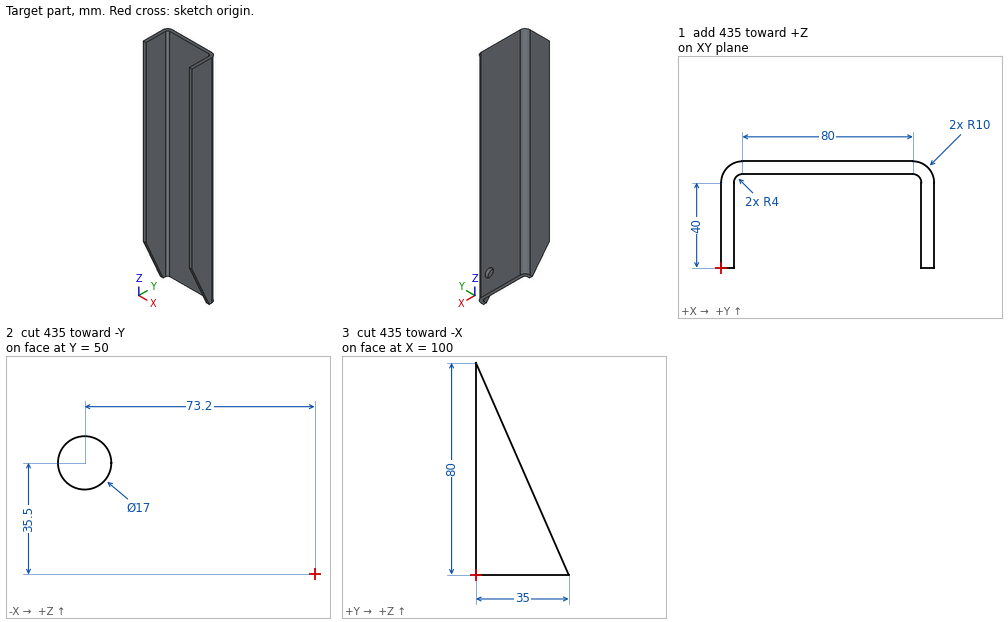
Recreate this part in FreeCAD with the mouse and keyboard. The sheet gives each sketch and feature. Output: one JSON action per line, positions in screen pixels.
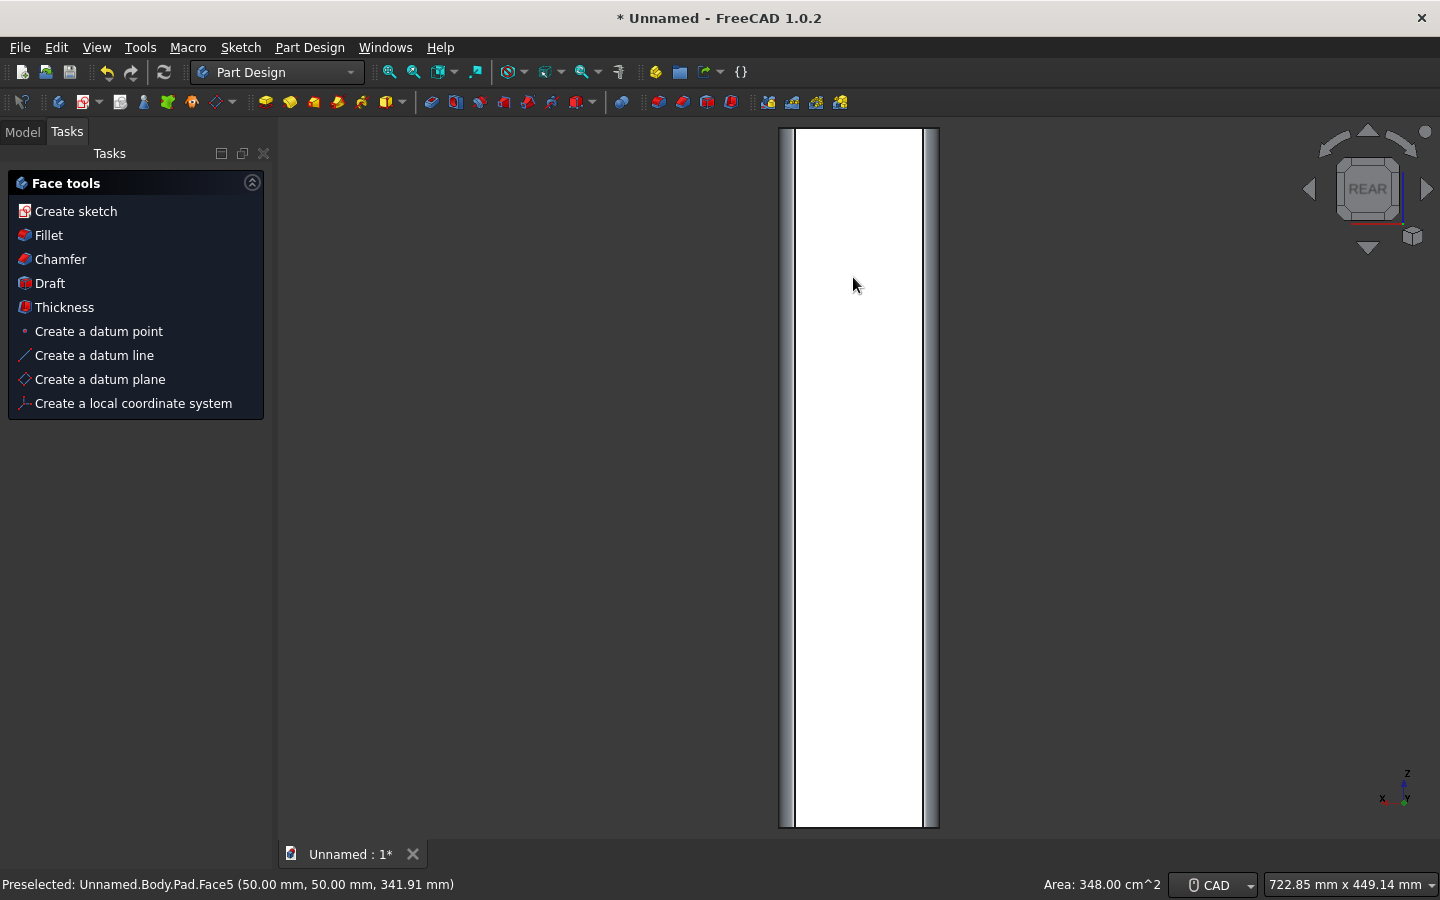
{"action": "left_click", "coordinate": [84, 102]}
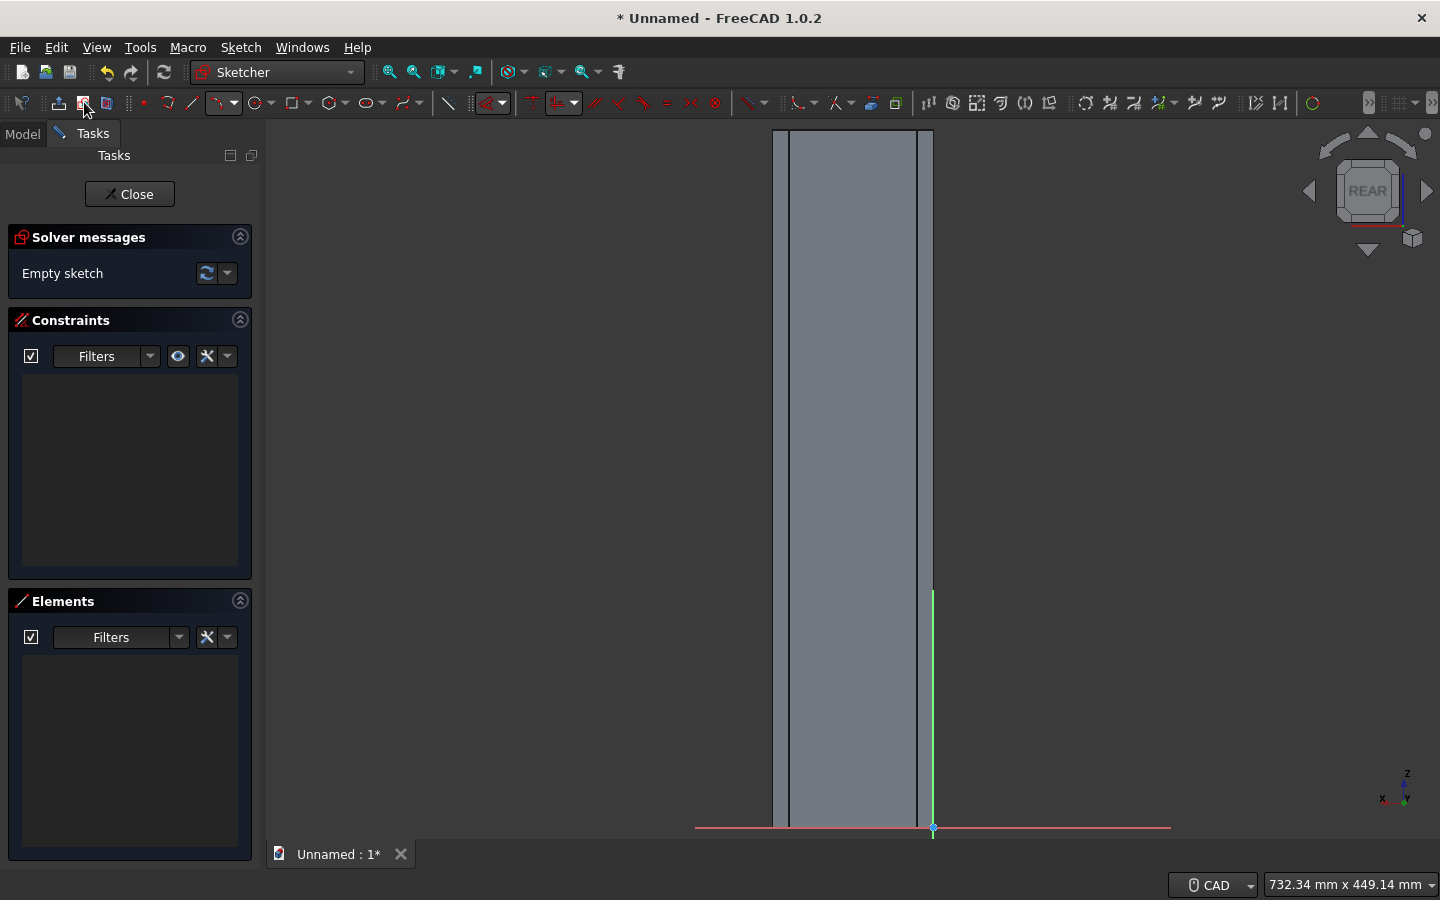
{"action": "scroll", "coordinate": [818, 790], "scroll_direction": "up", "scroll_amount": 14}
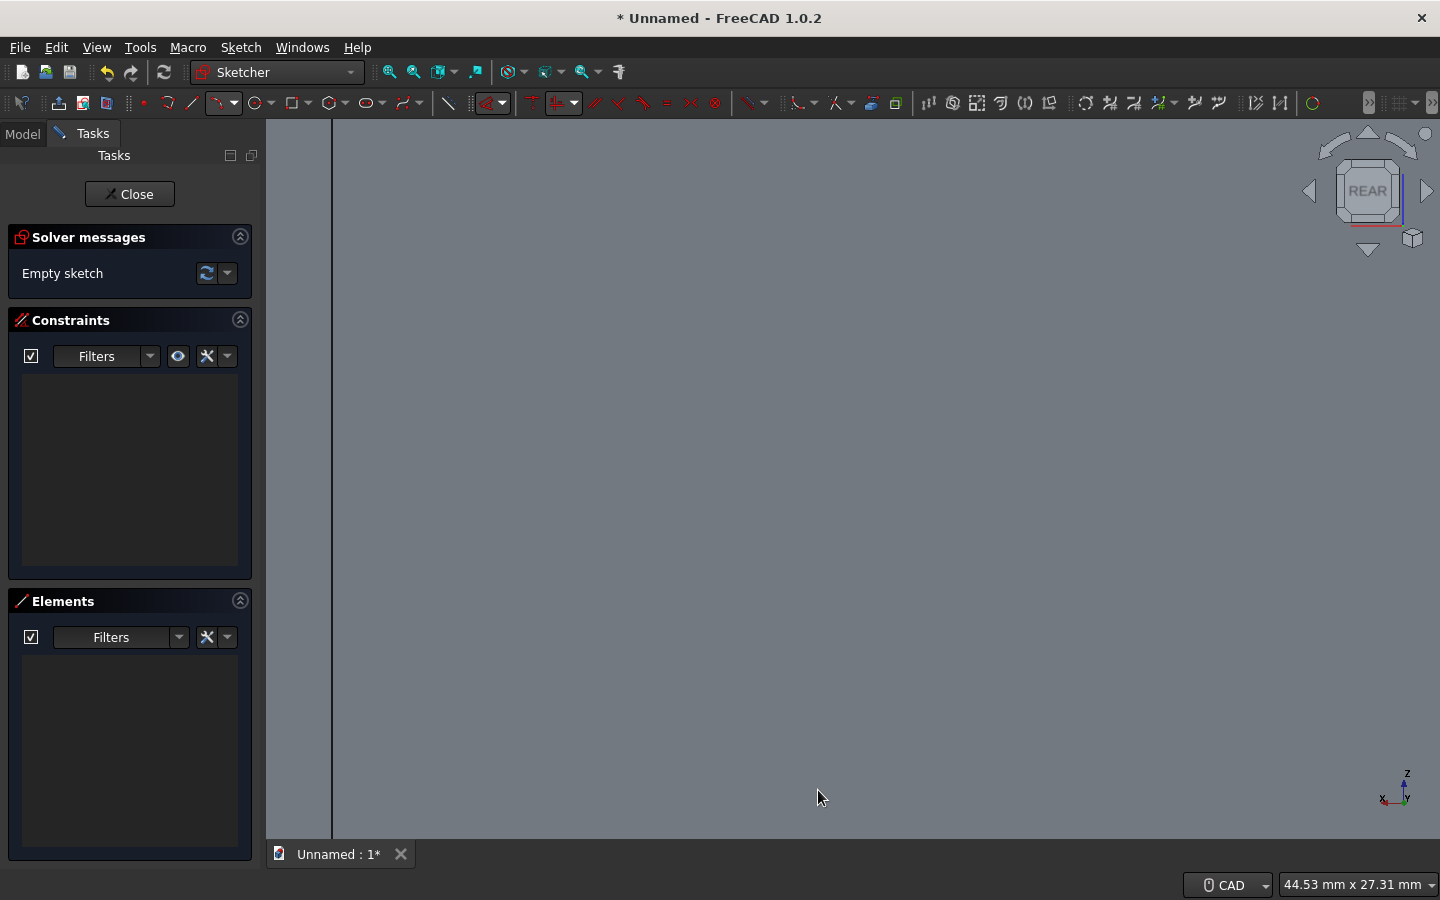
{"action": "left_click", "coordinate": [256, 104]}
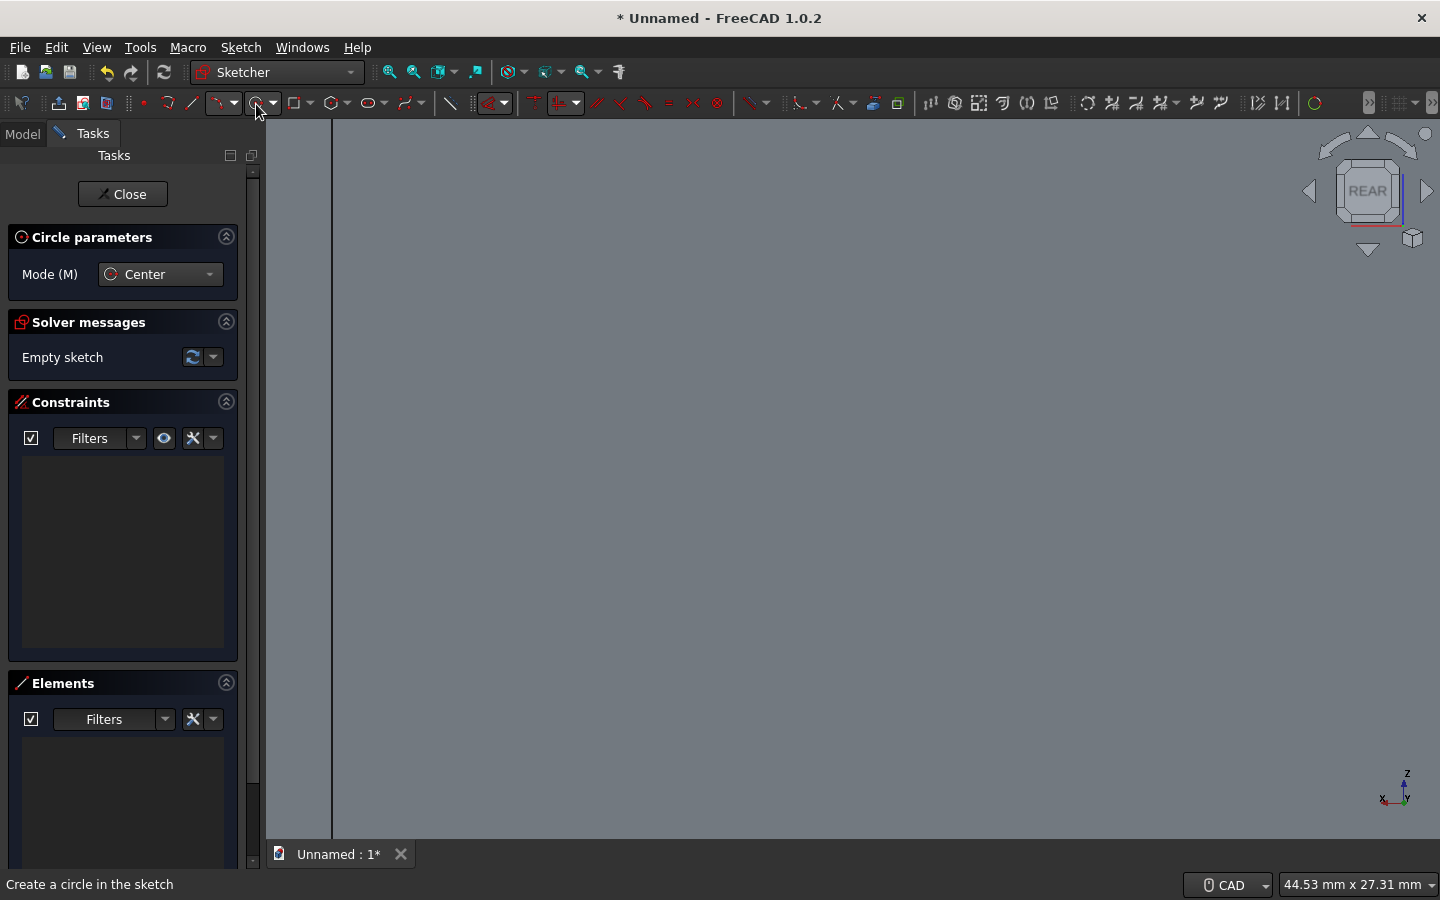
{"action": "left_click", "coordinate": [775, 459]}
{"action": "mouse_move", "coordinate": [933, 301]}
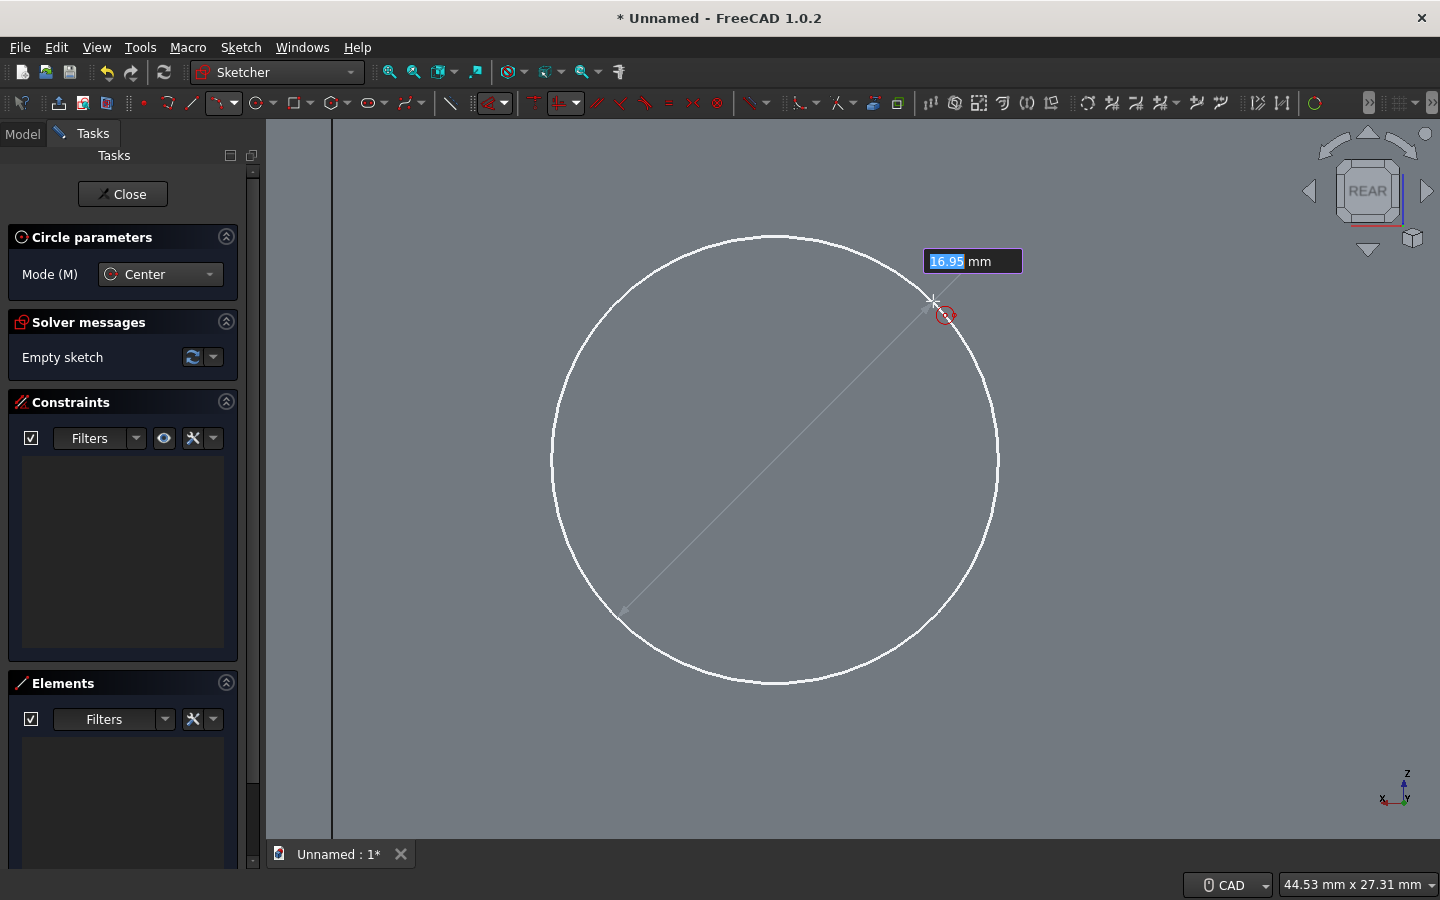
{"action": "type", "text": "17"}
{"action": "key", "text": "Return"}
{"action": "key", "text": "Escape"}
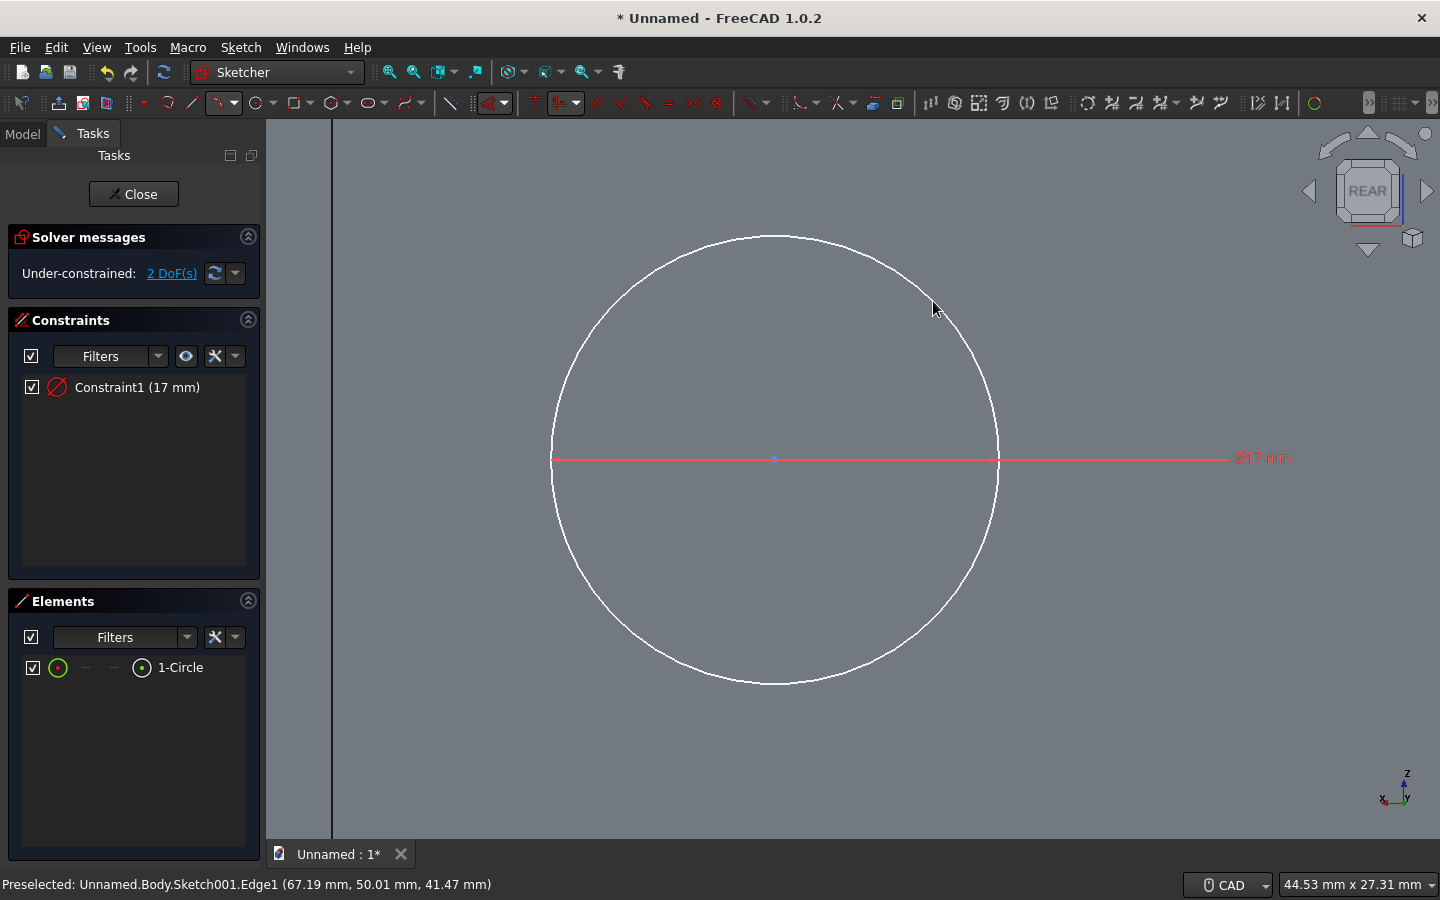
{"action": "left_click", "coordinate": [775, 460]}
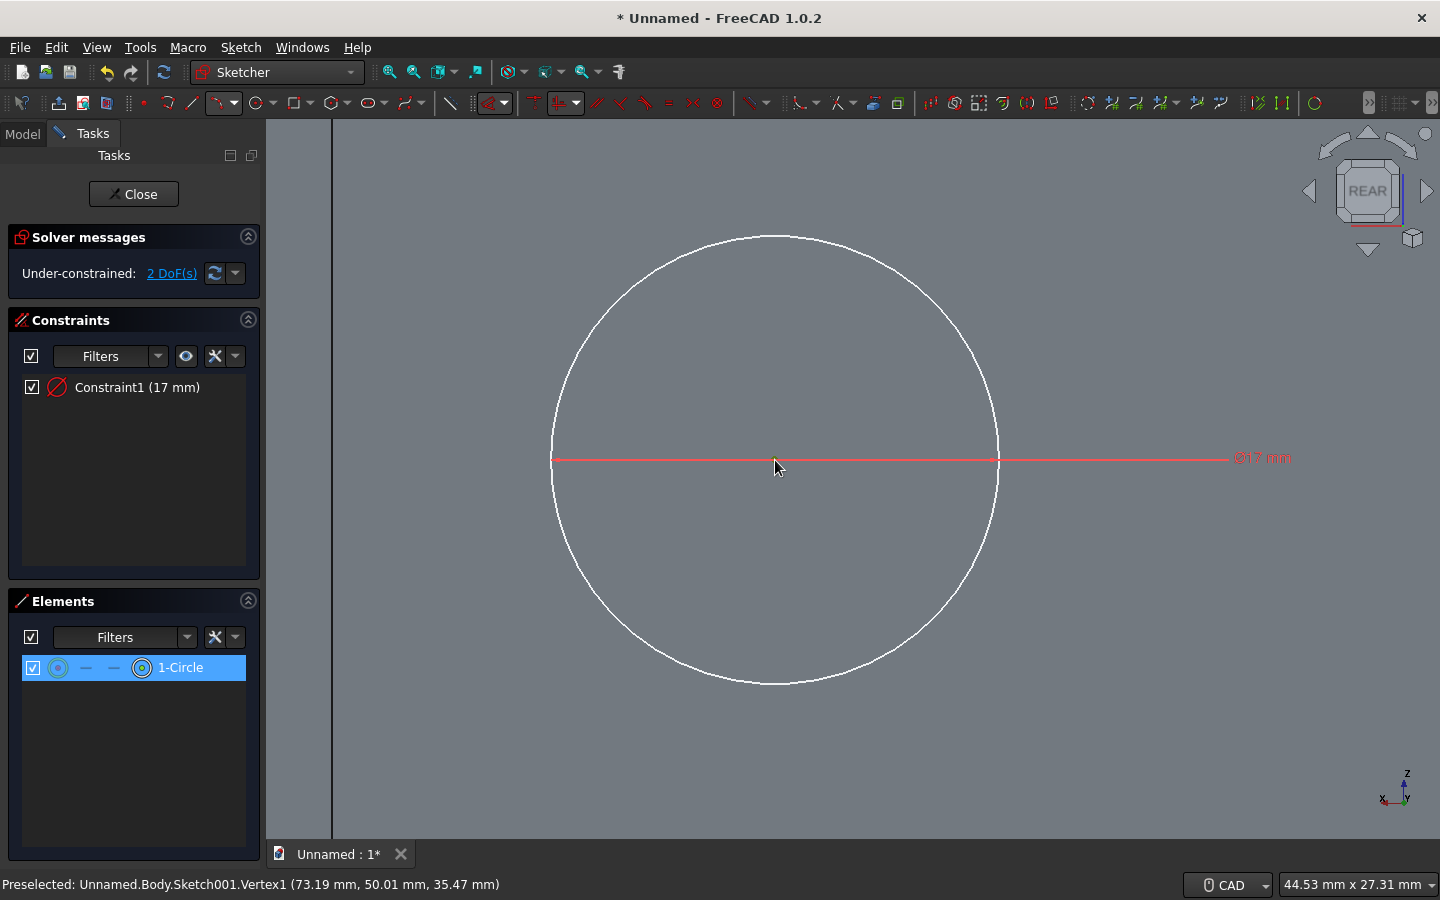
{"action": "left_click", "coordinate": [506, 104]}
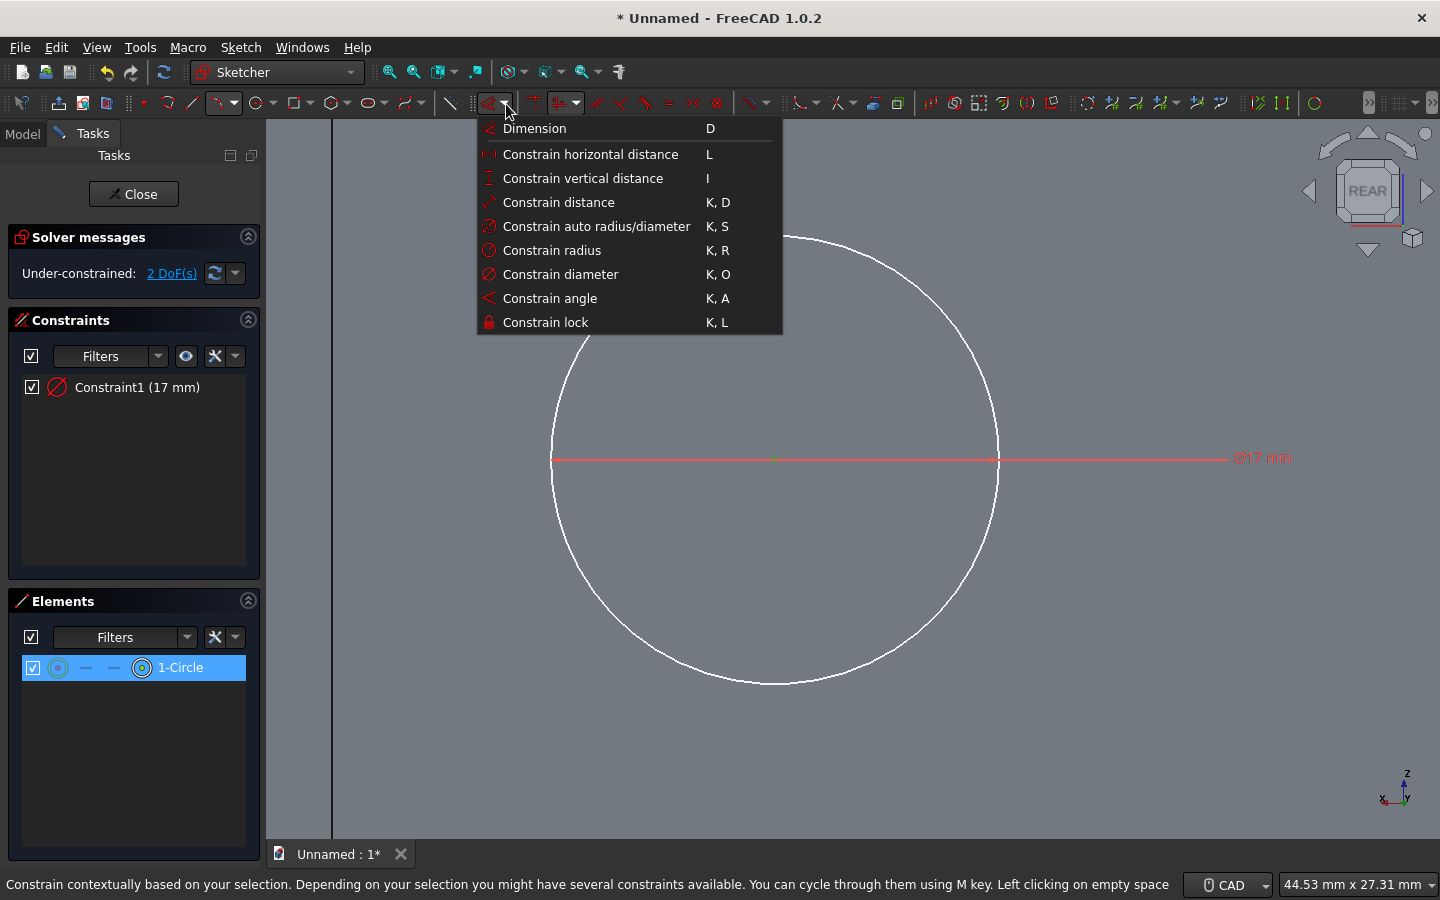
{"action": "left_click", "coordinate": [630, 154]}